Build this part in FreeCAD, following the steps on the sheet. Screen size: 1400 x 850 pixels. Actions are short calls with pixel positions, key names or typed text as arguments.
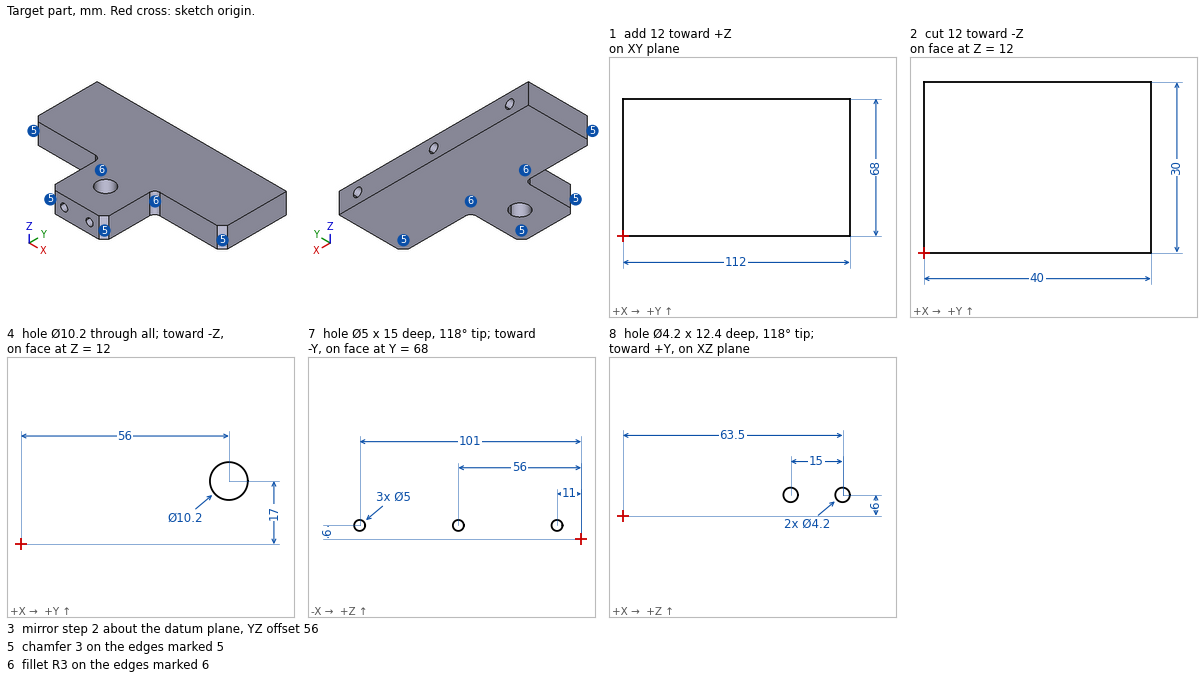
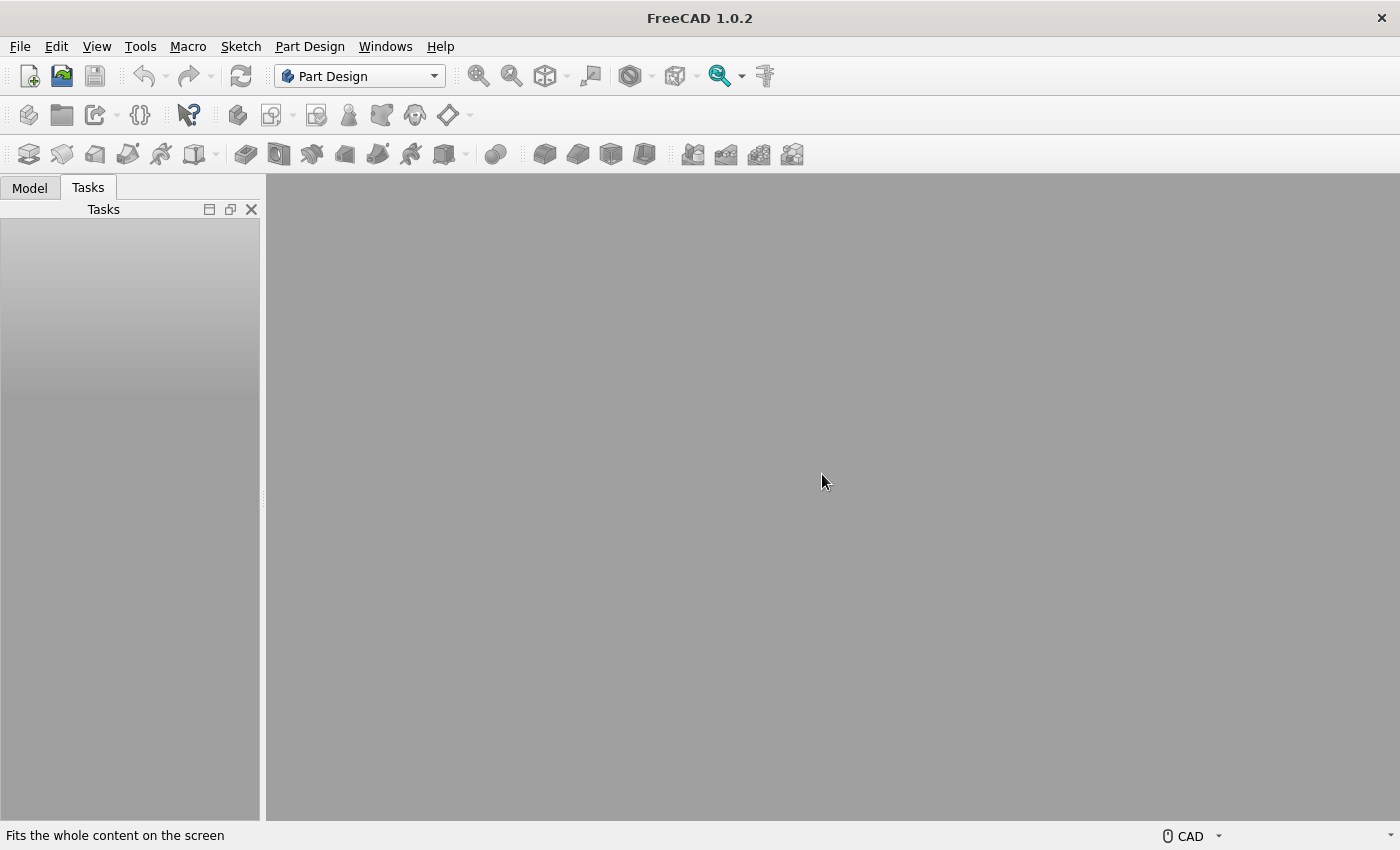
click(29, 76)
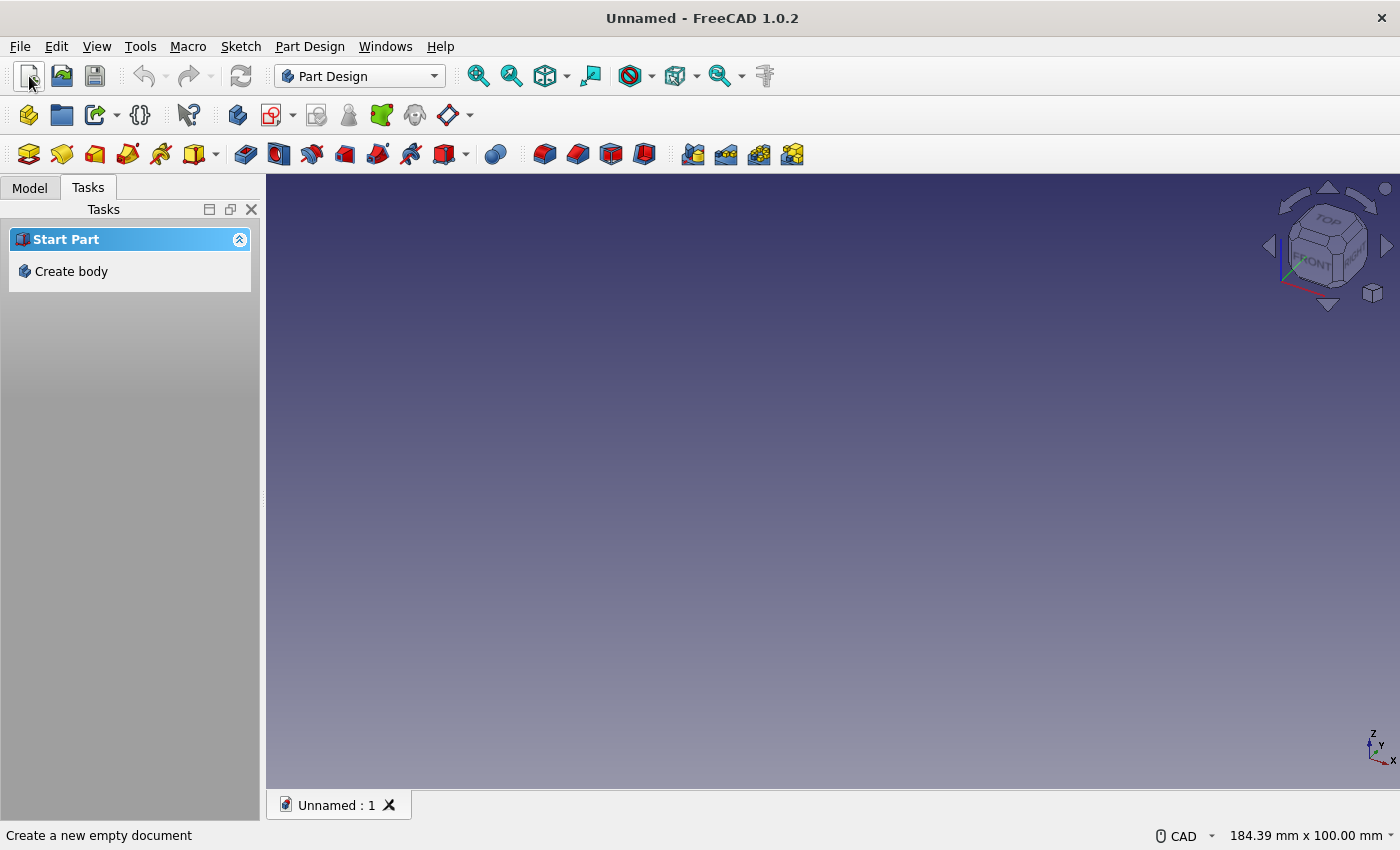
click(270, 116)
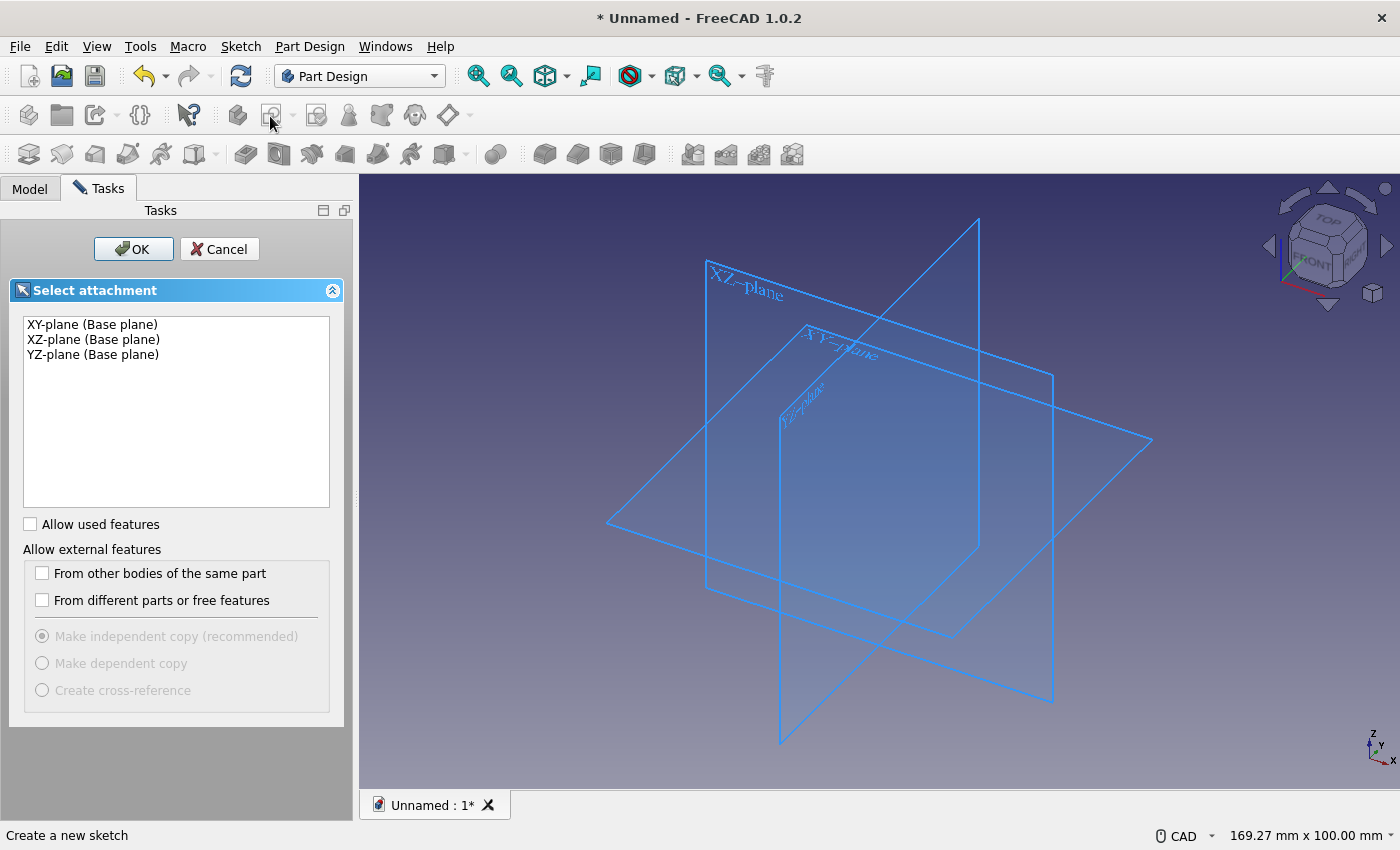
click(84, 324)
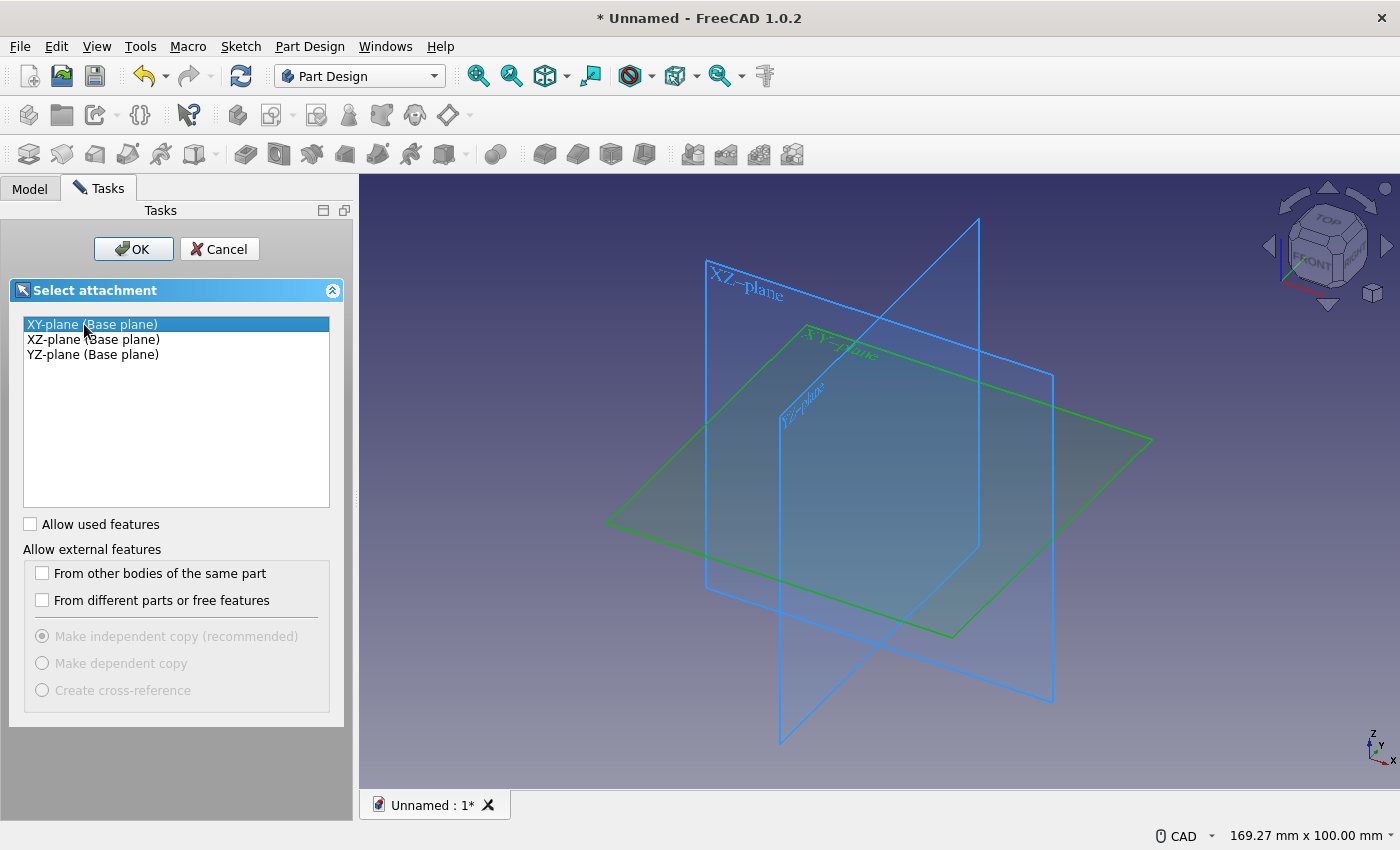
click(134, 249)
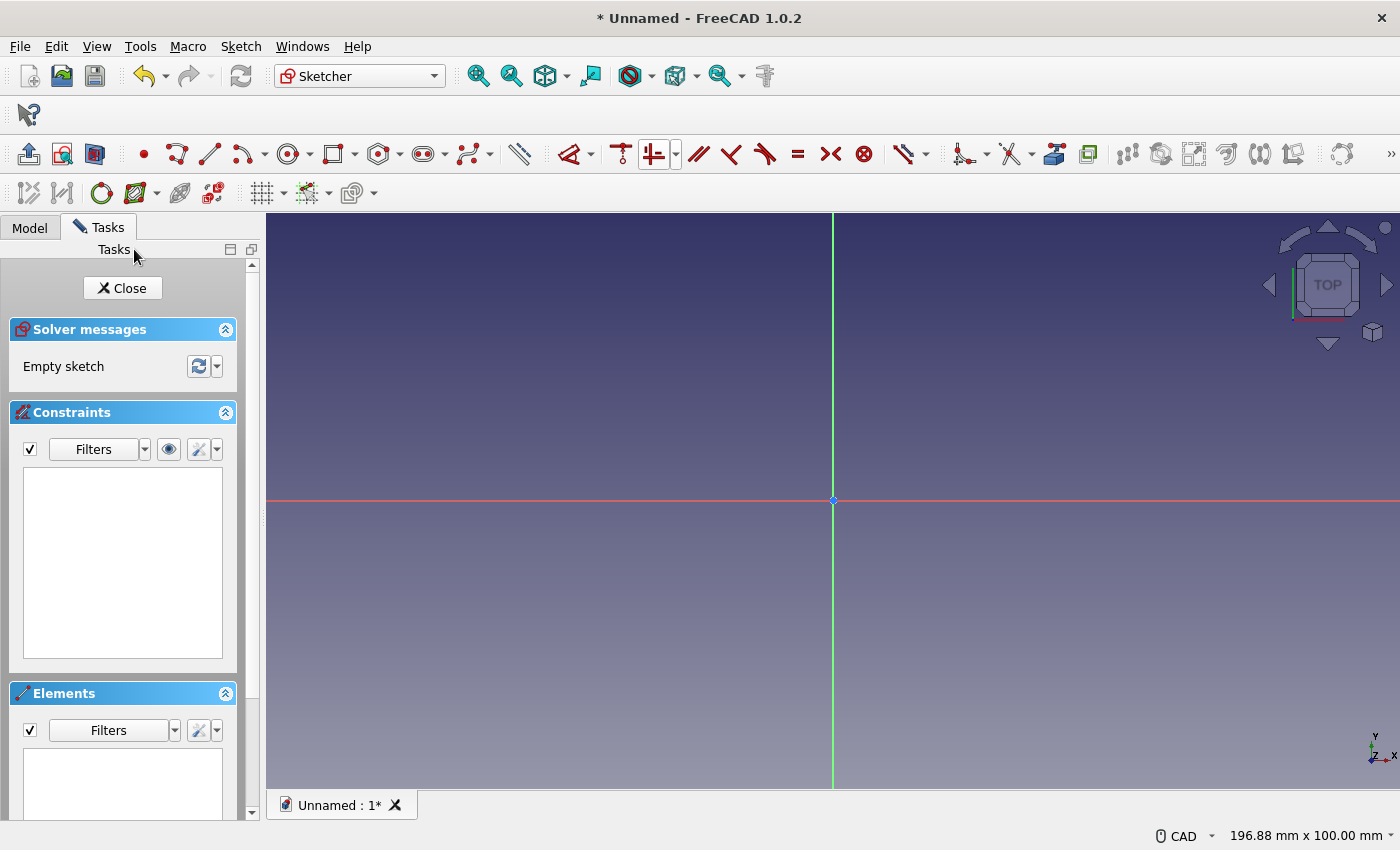
scroll(294, 761, down, 2)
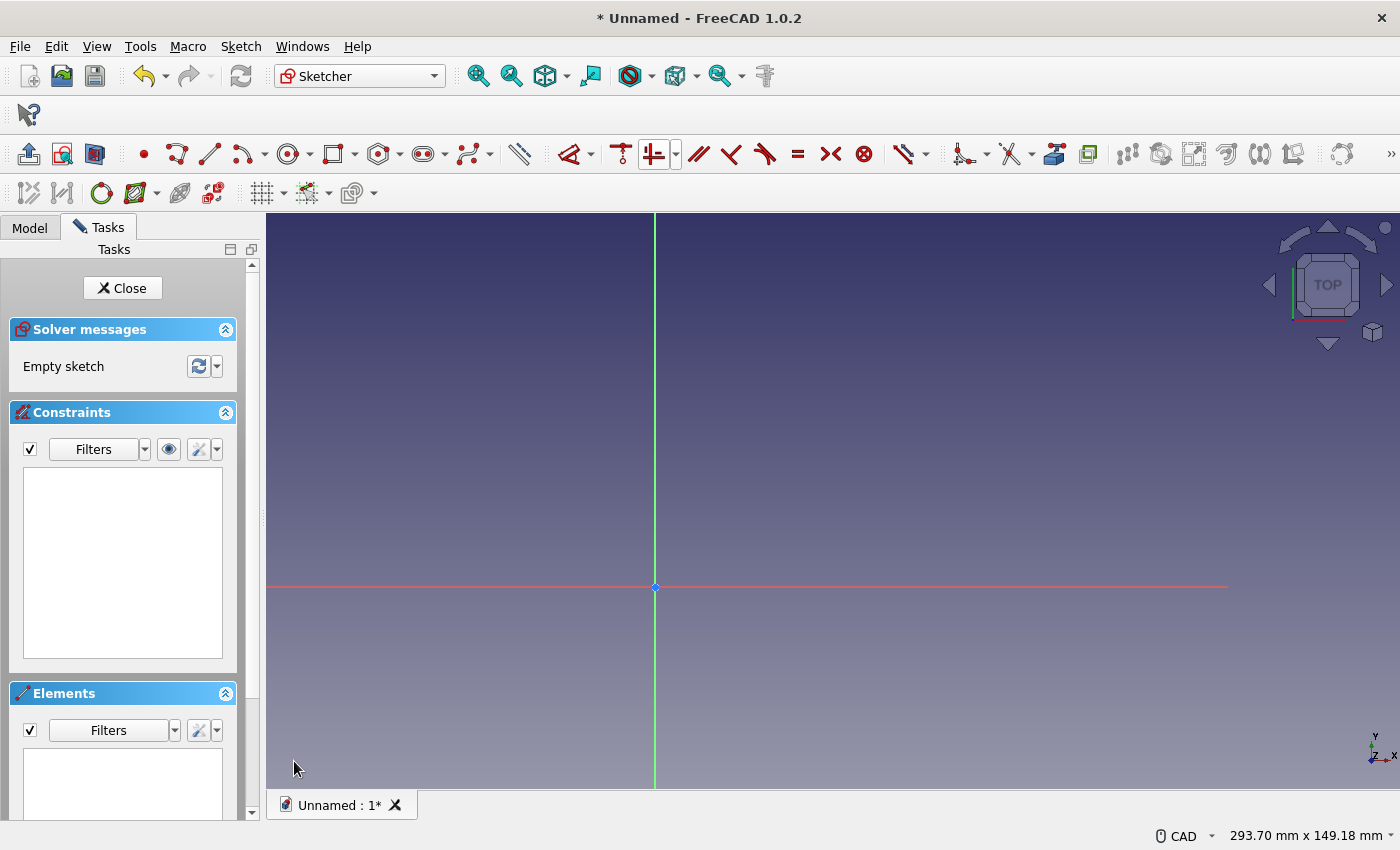
scroll(1089, 364, up, 2)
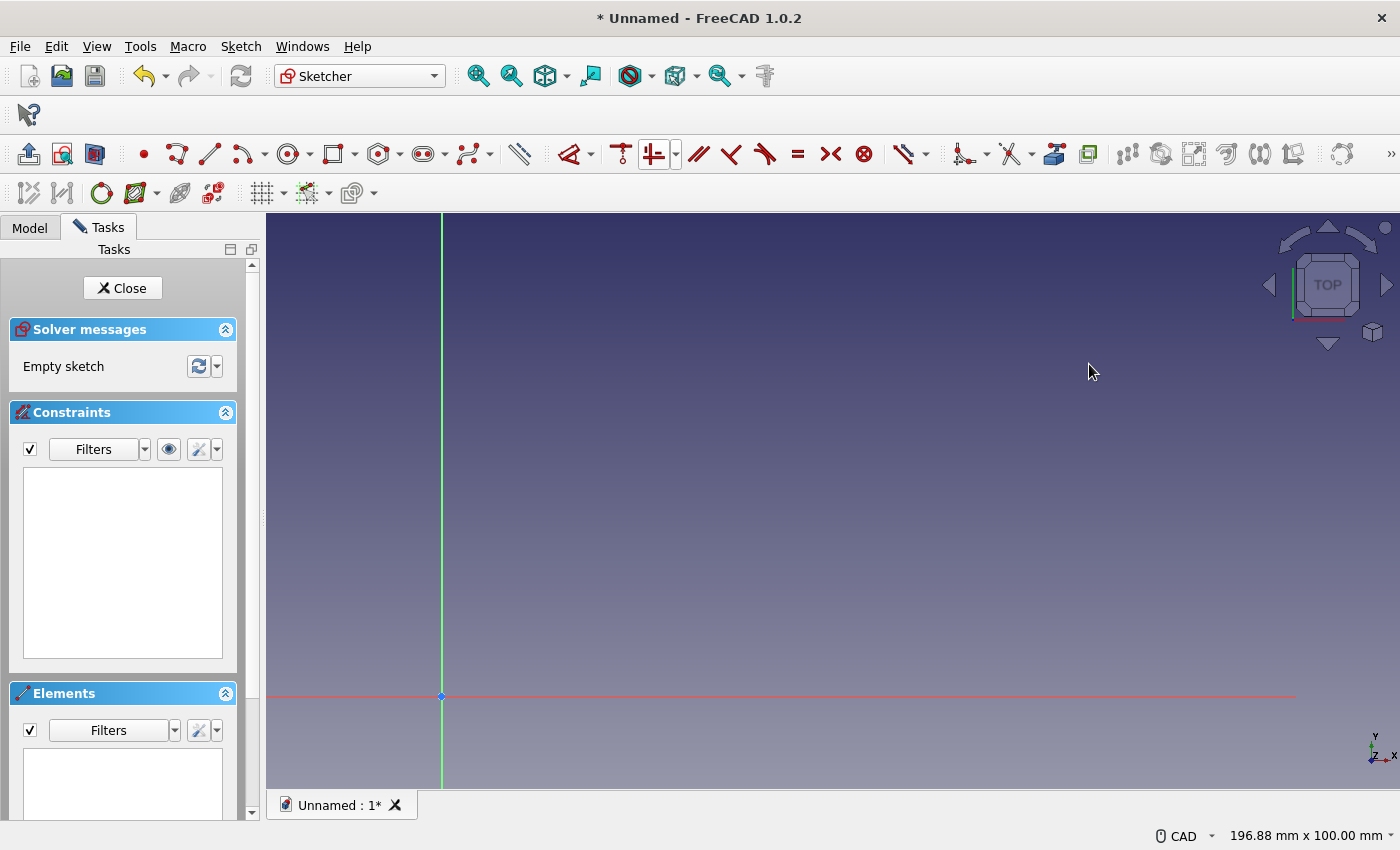
click(332, 154)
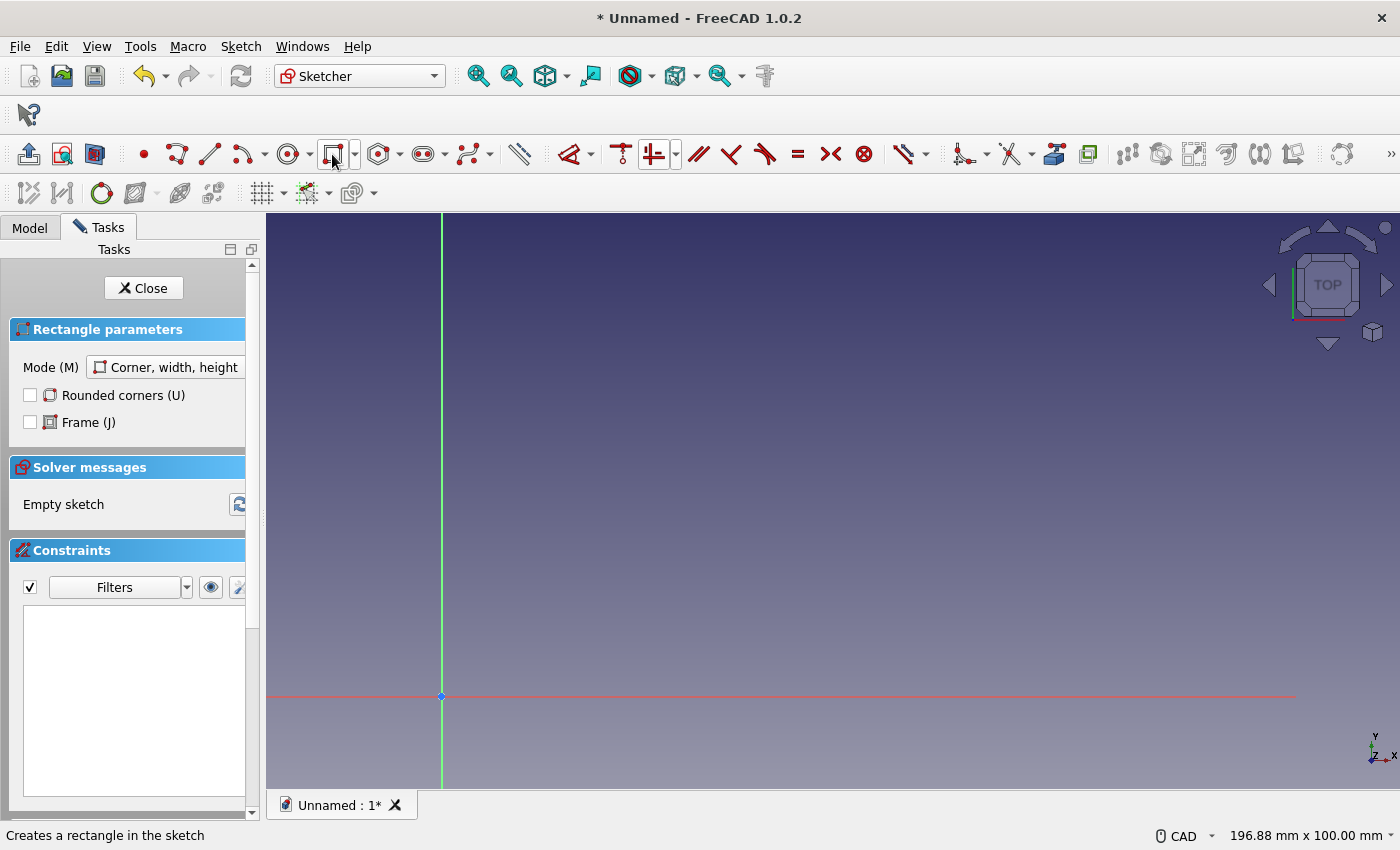
click(442, 697)
click(1087, 305)
key(Escape)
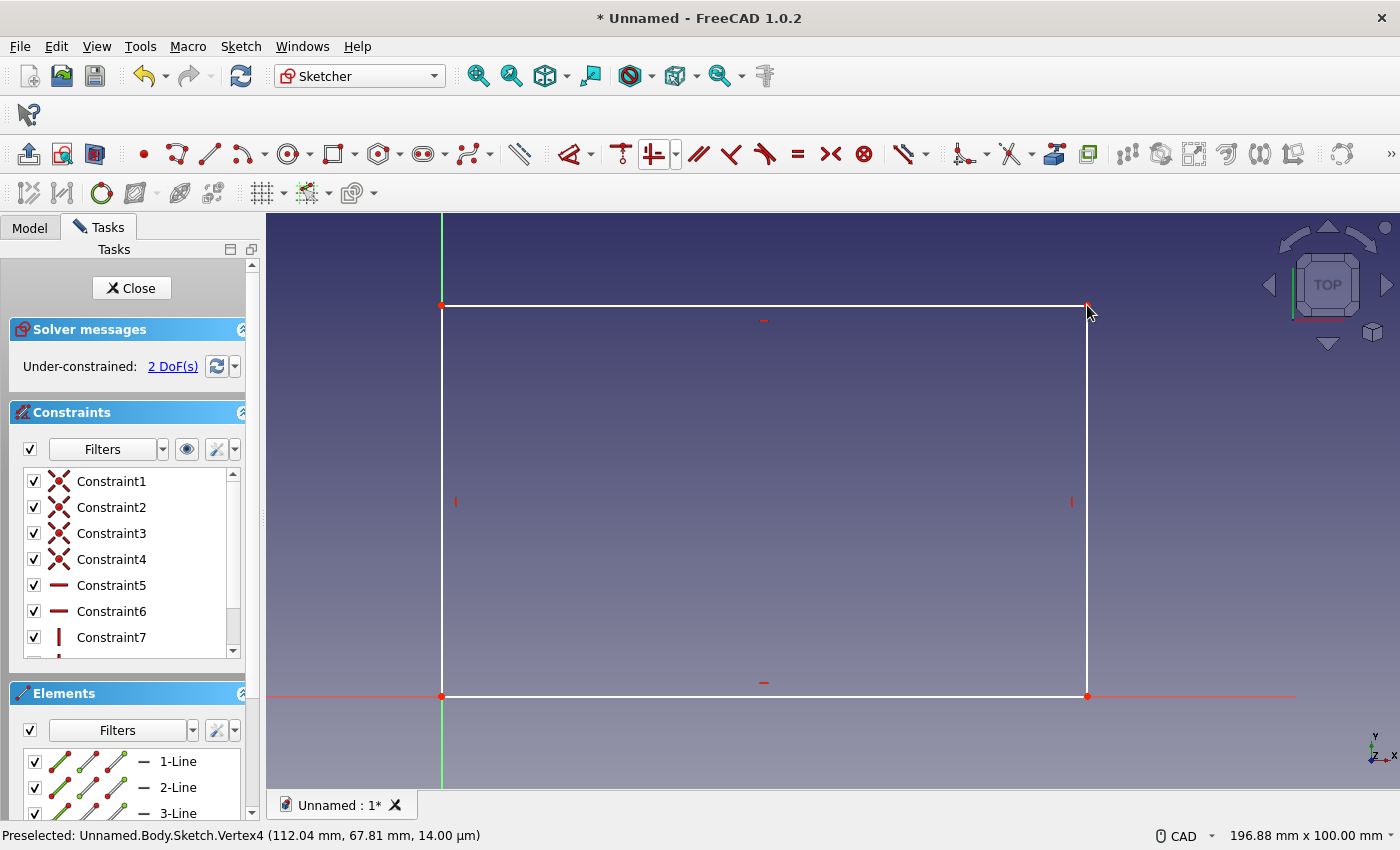
click(568, 154)